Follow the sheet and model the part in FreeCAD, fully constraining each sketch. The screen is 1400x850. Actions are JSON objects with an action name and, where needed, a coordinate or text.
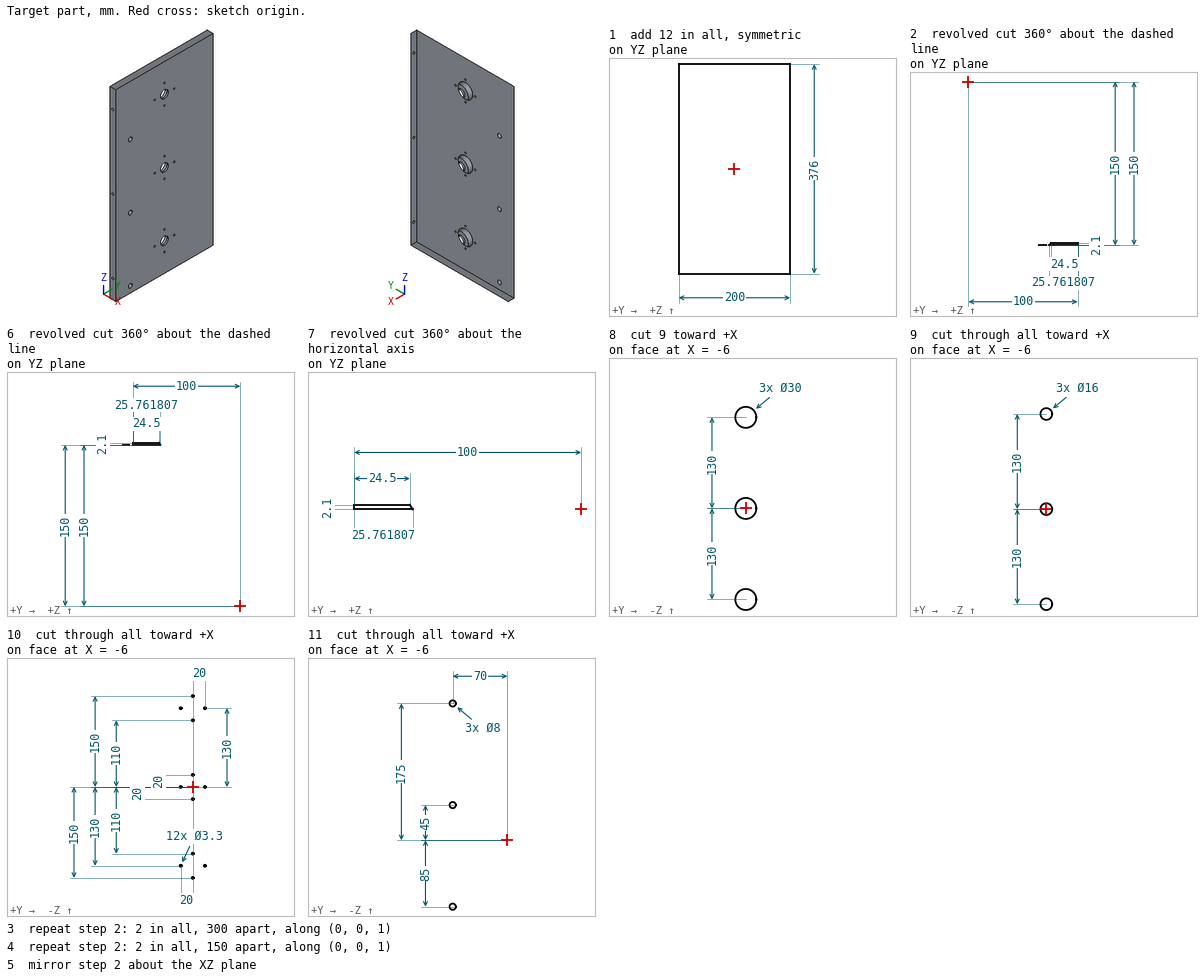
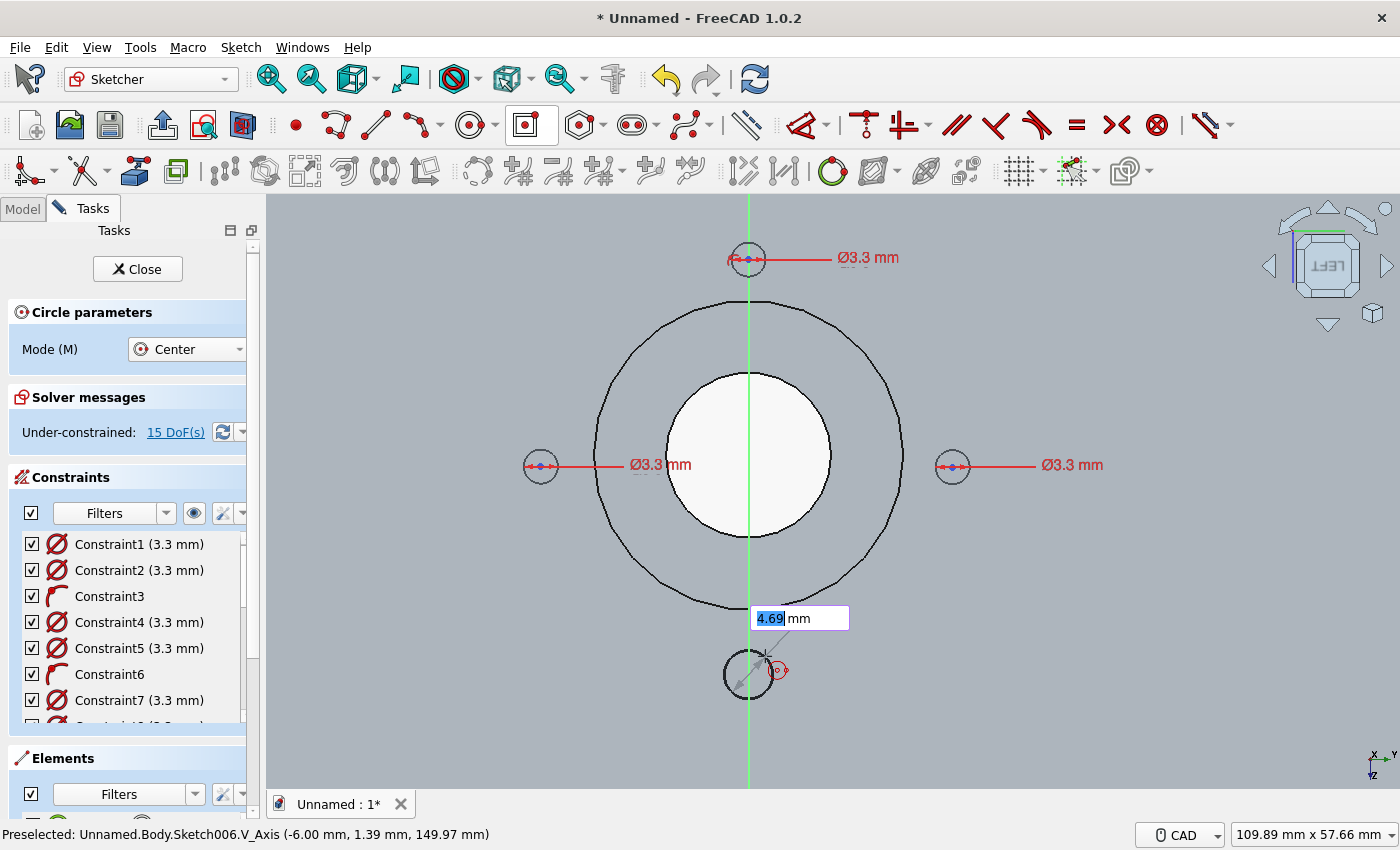
{"action": "type", "text": "3.3"}
{"action": "key", "text": "Return"}
{"action": "key", "text": "Escape"}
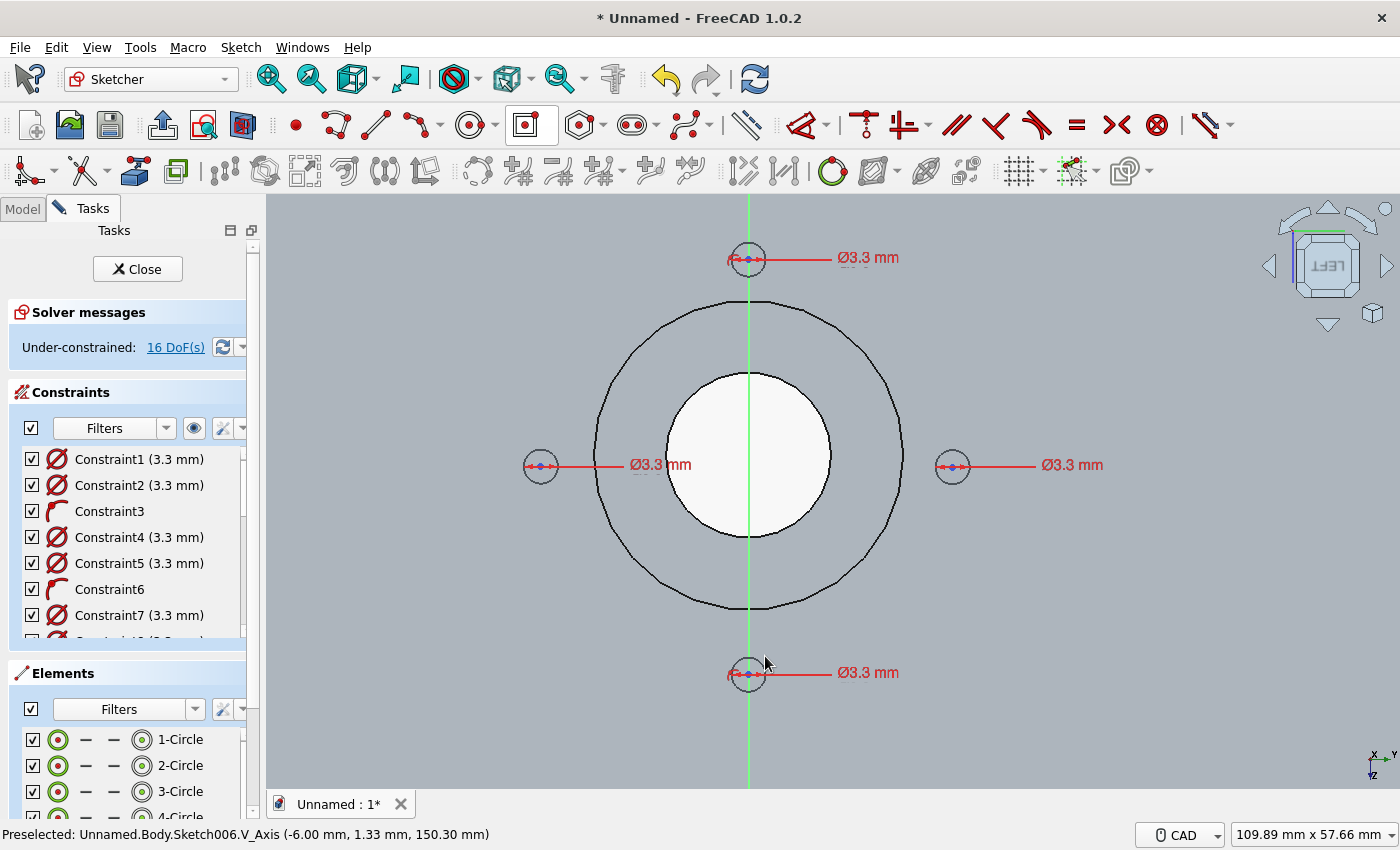
{"action": "scroll", "coordinate": [766, 663], "scroll_direction": "down", "scroll_amount": 11}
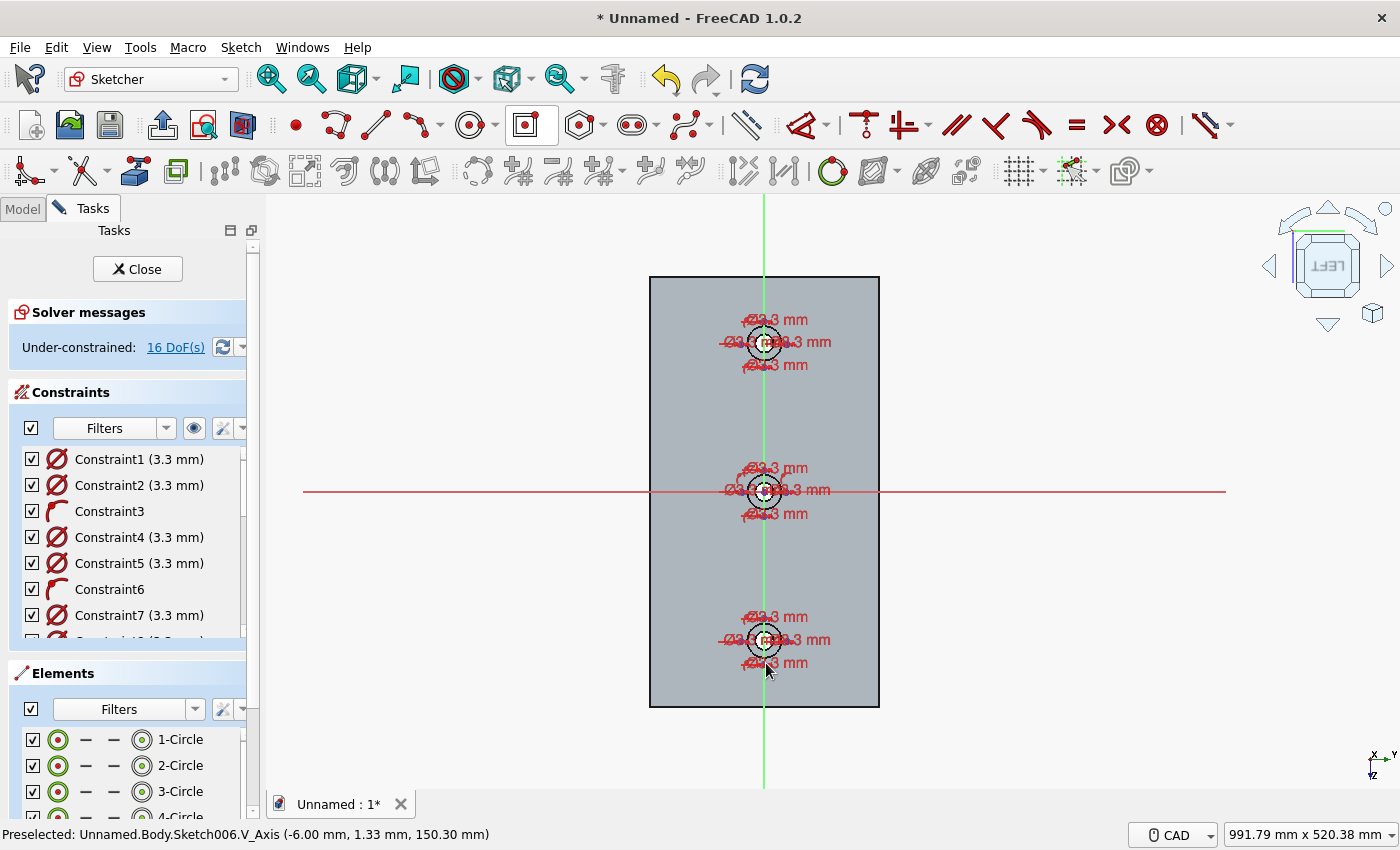
{"action": "left_click", "coordinate": [741, 642]}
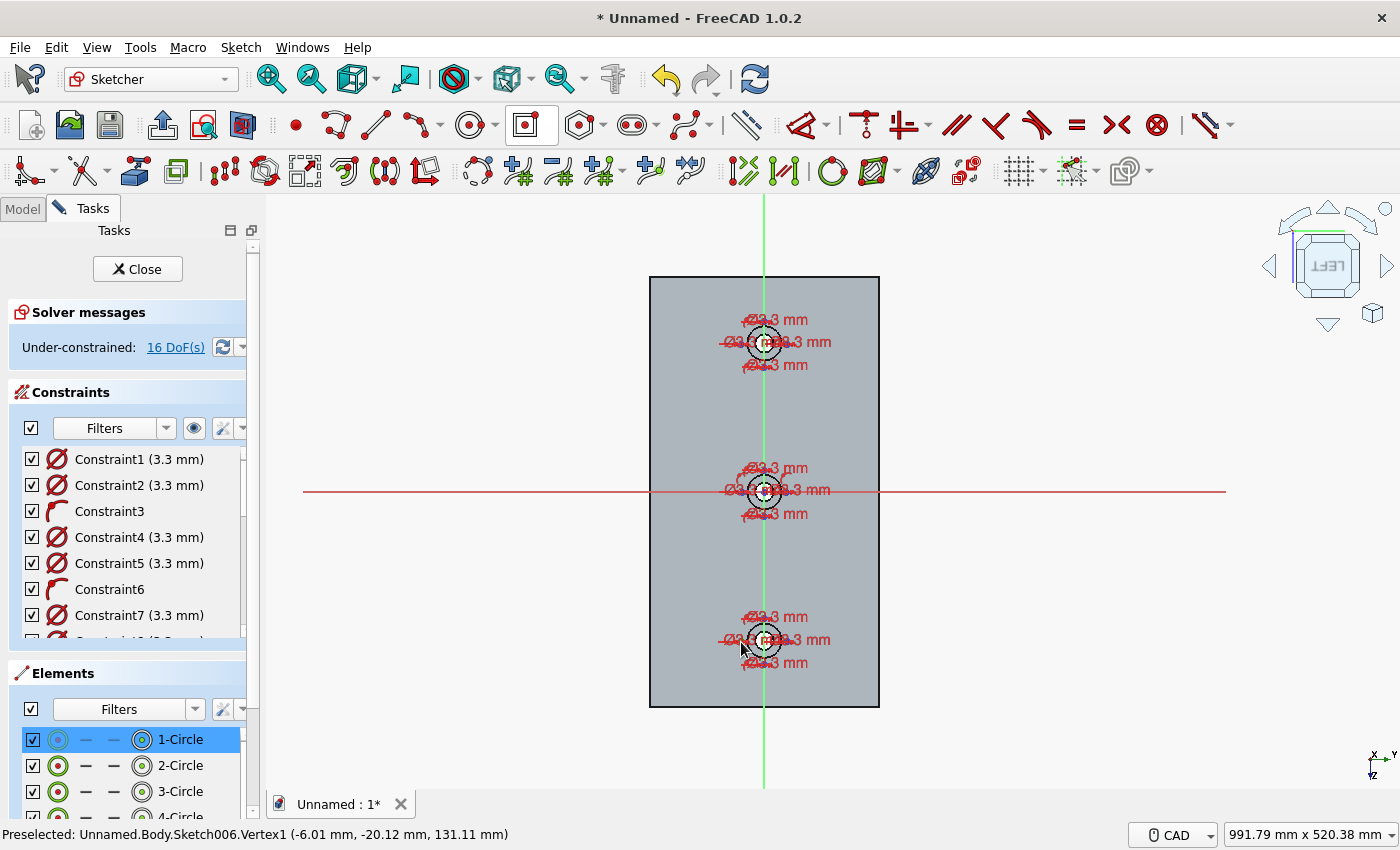
{"action": "left_click", "coordinate": [742, 344]}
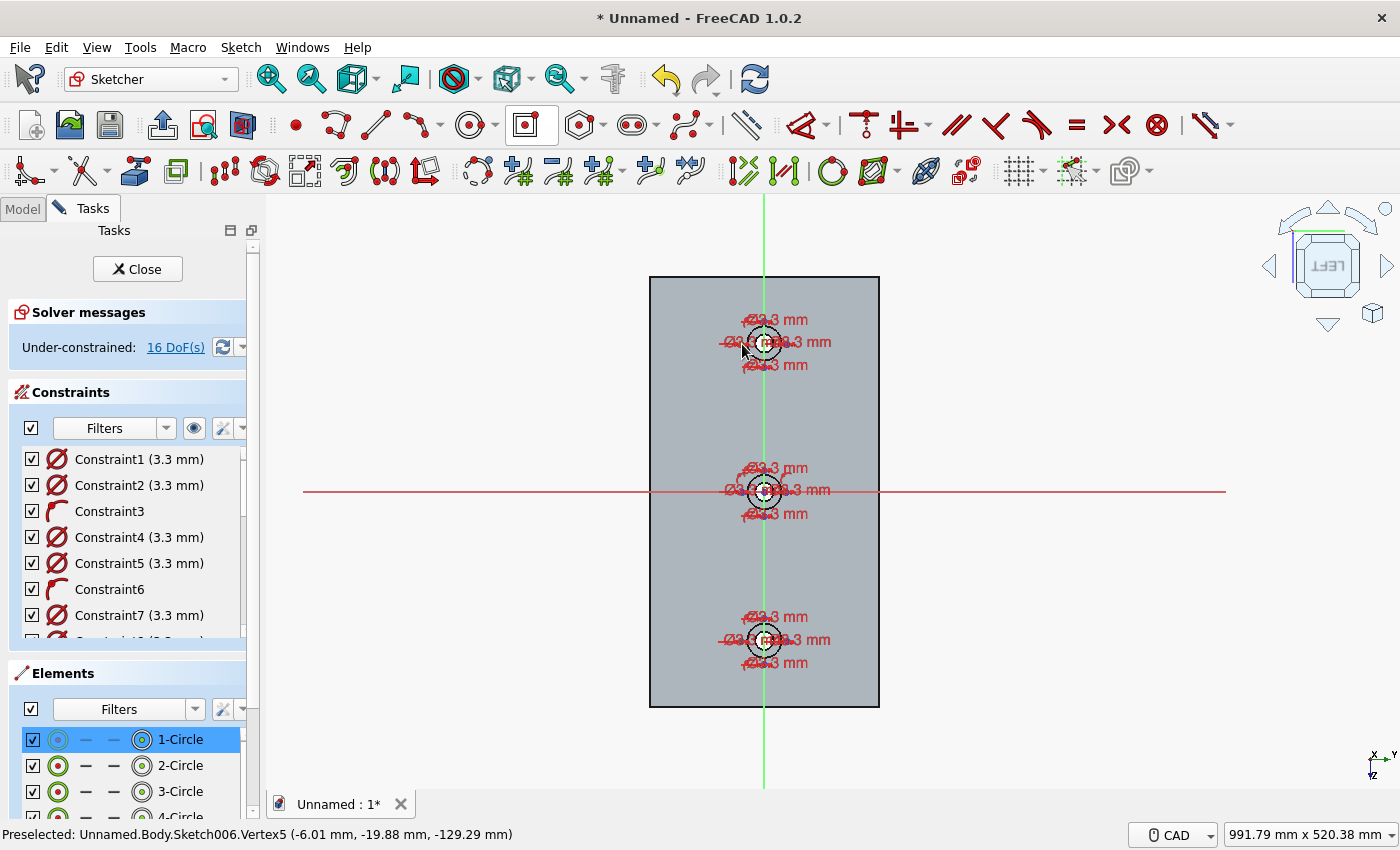
{"action": "left_click", "coordinate": [930, 126]}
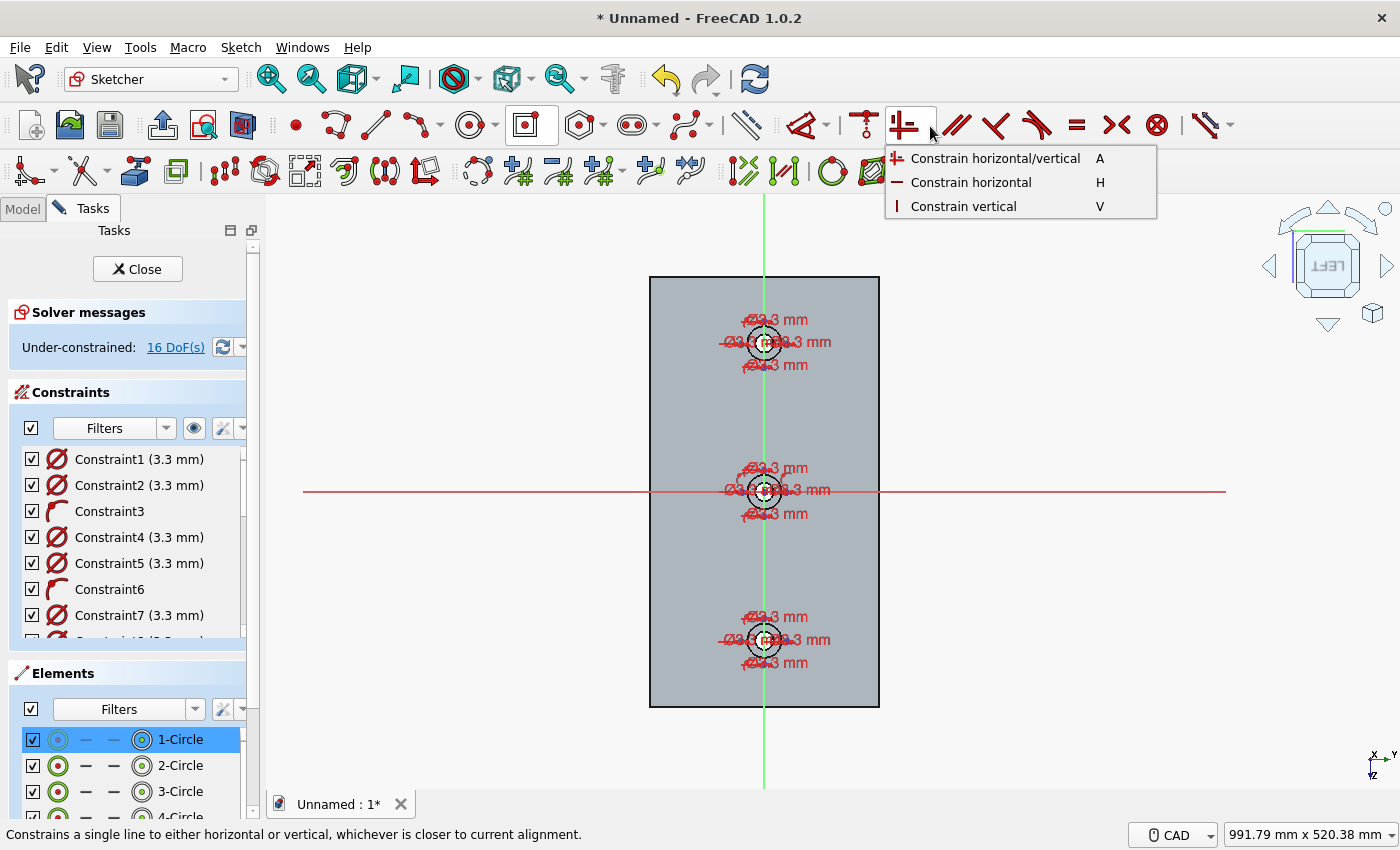
{"action": "left_click", "coordinate": [1021, 206]}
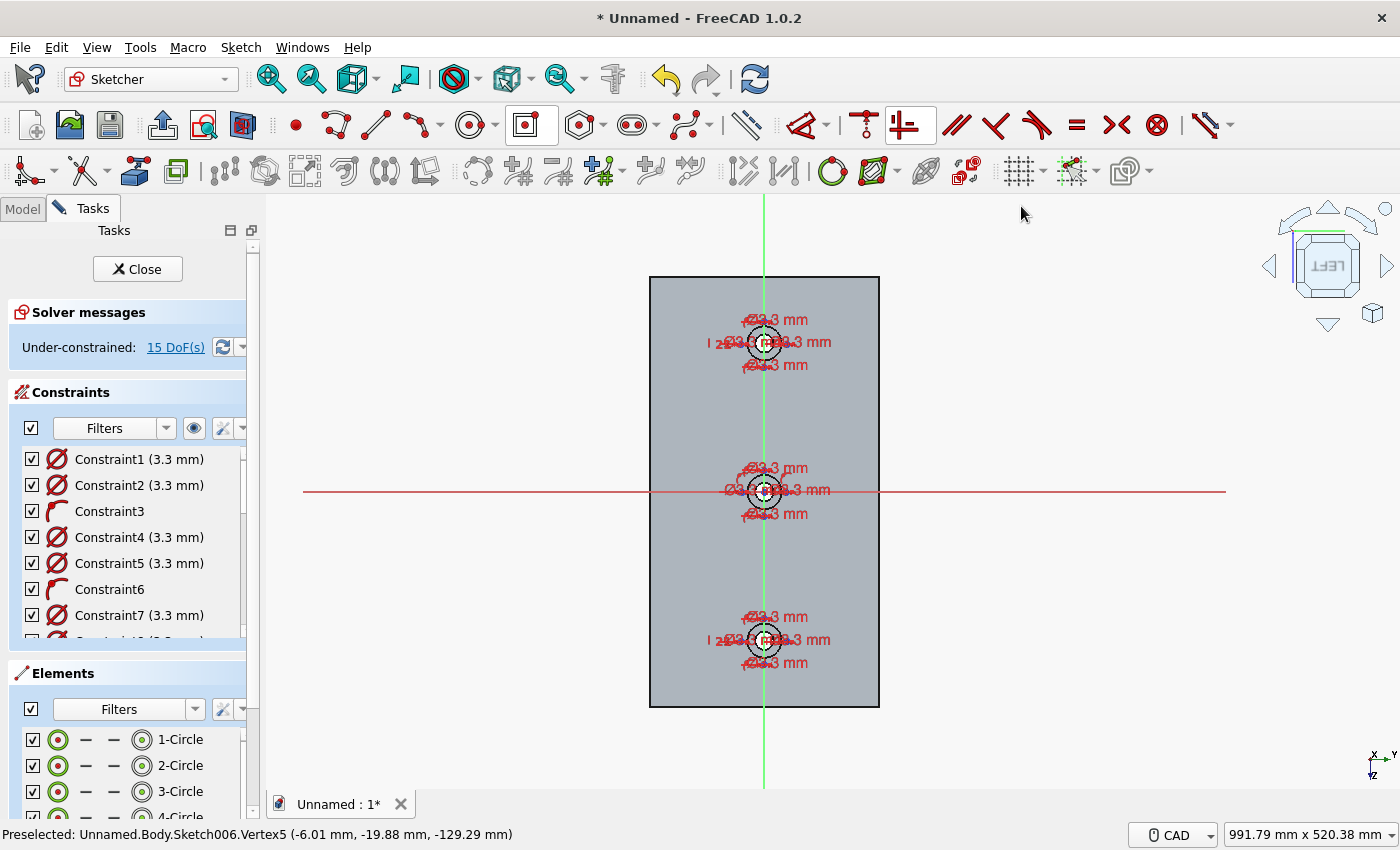
{"action": "left_click", "coordinate": [788, 344]}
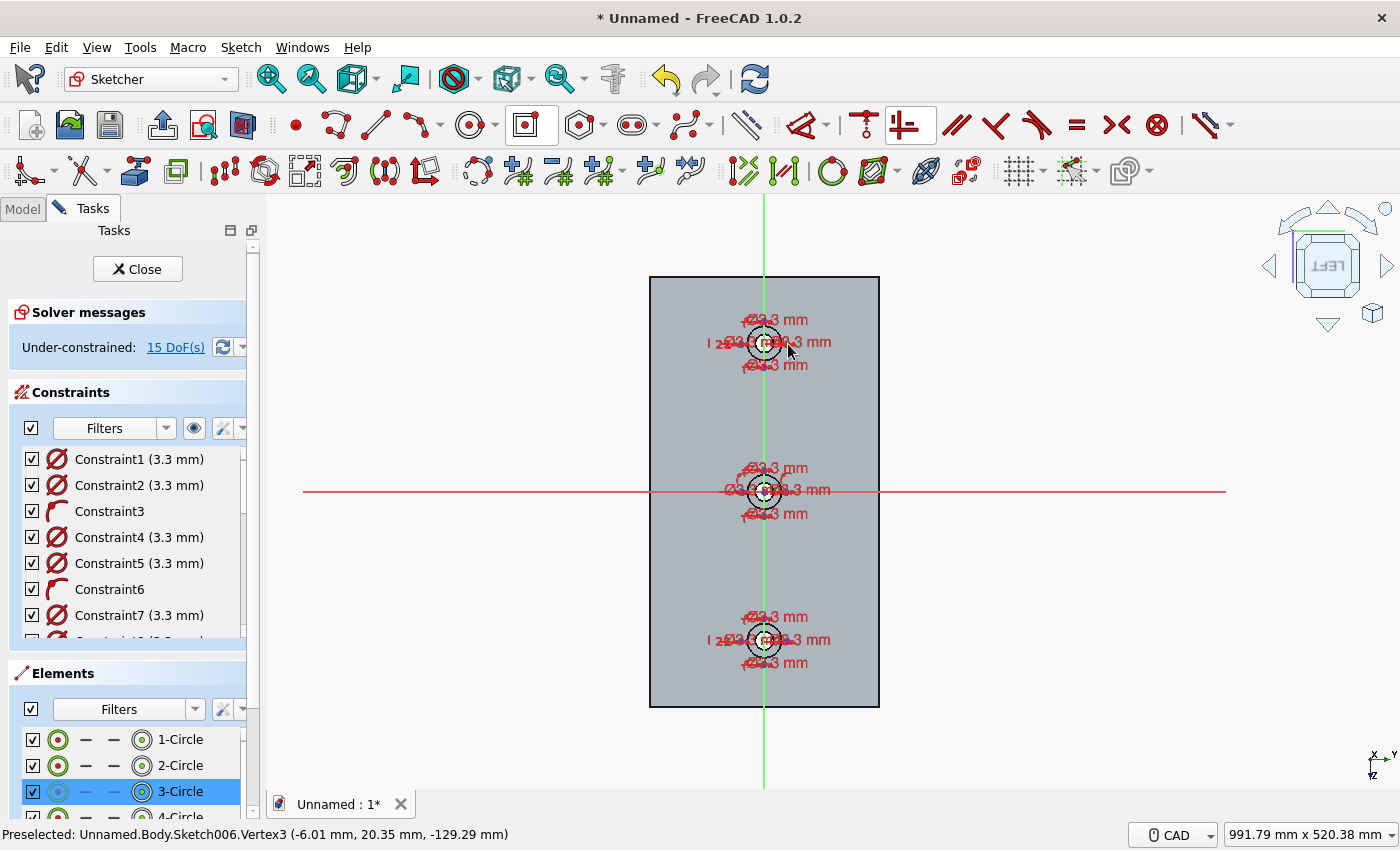
{"action": "left_click", "coordinate": [741, 344]}